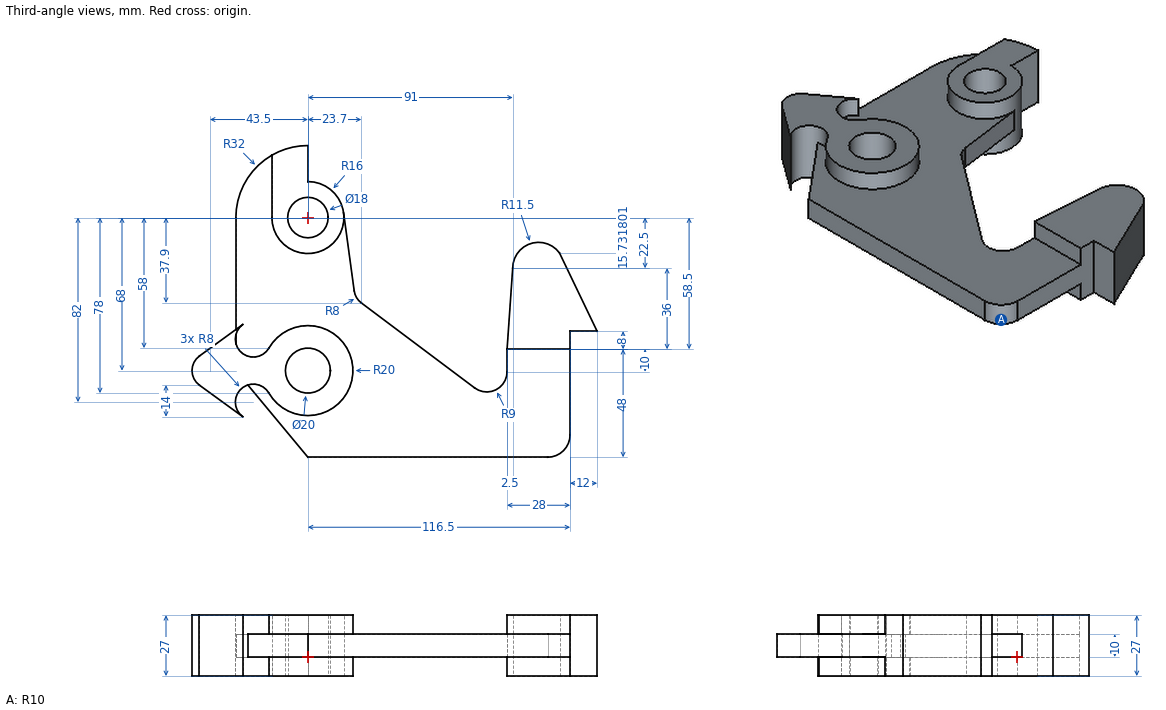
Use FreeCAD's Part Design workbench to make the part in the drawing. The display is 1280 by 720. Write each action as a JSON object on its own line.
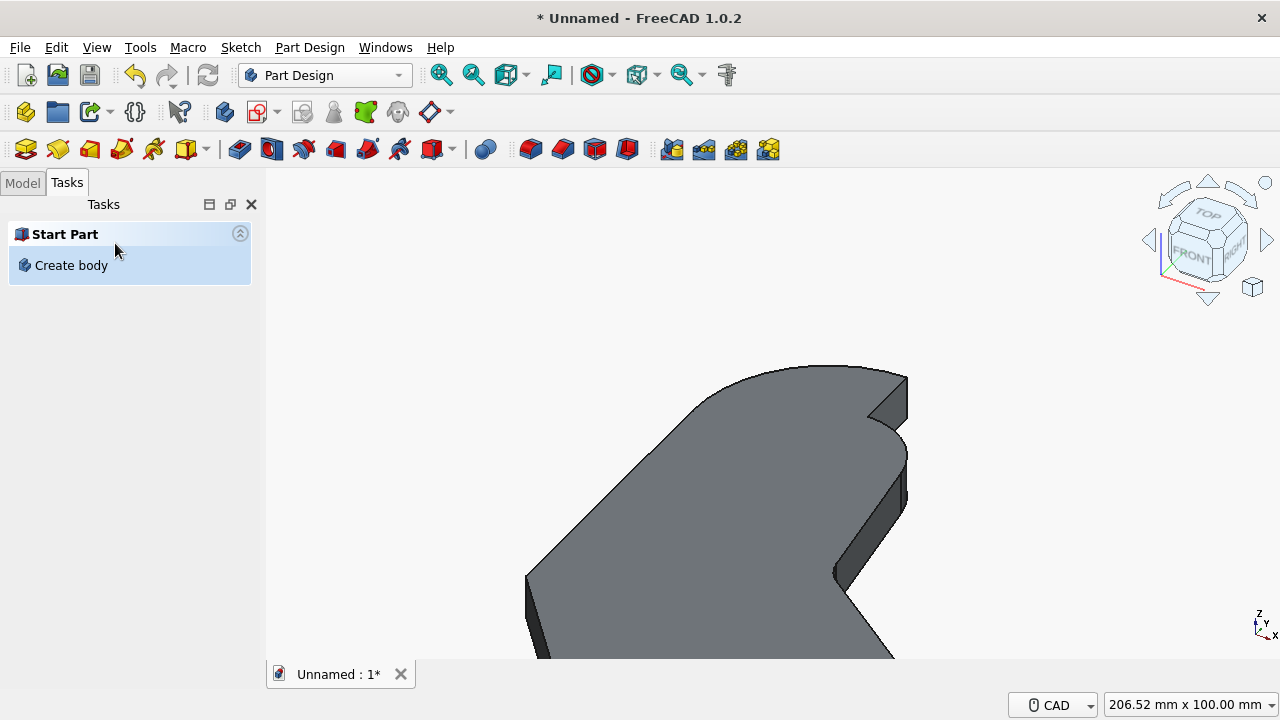
{"action": "left_click", "coordinate": [442, 76]}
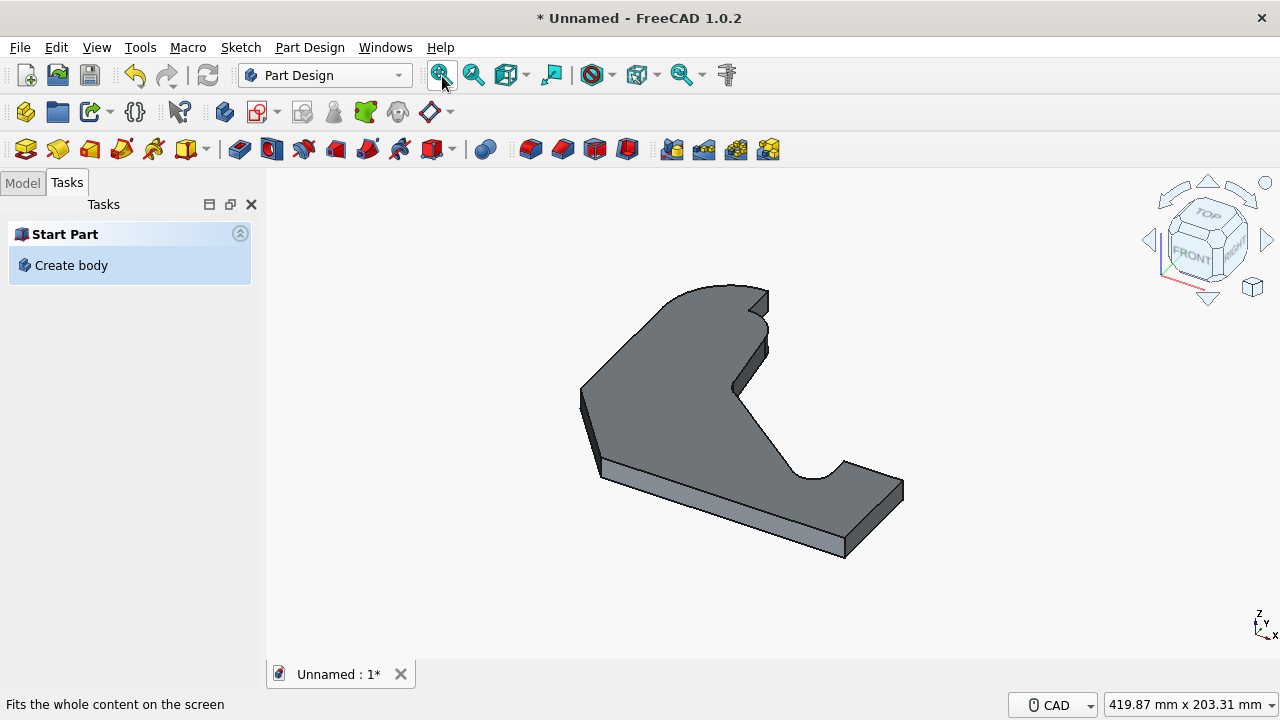
{"action": "left_click", "coordinate": [23, 182]}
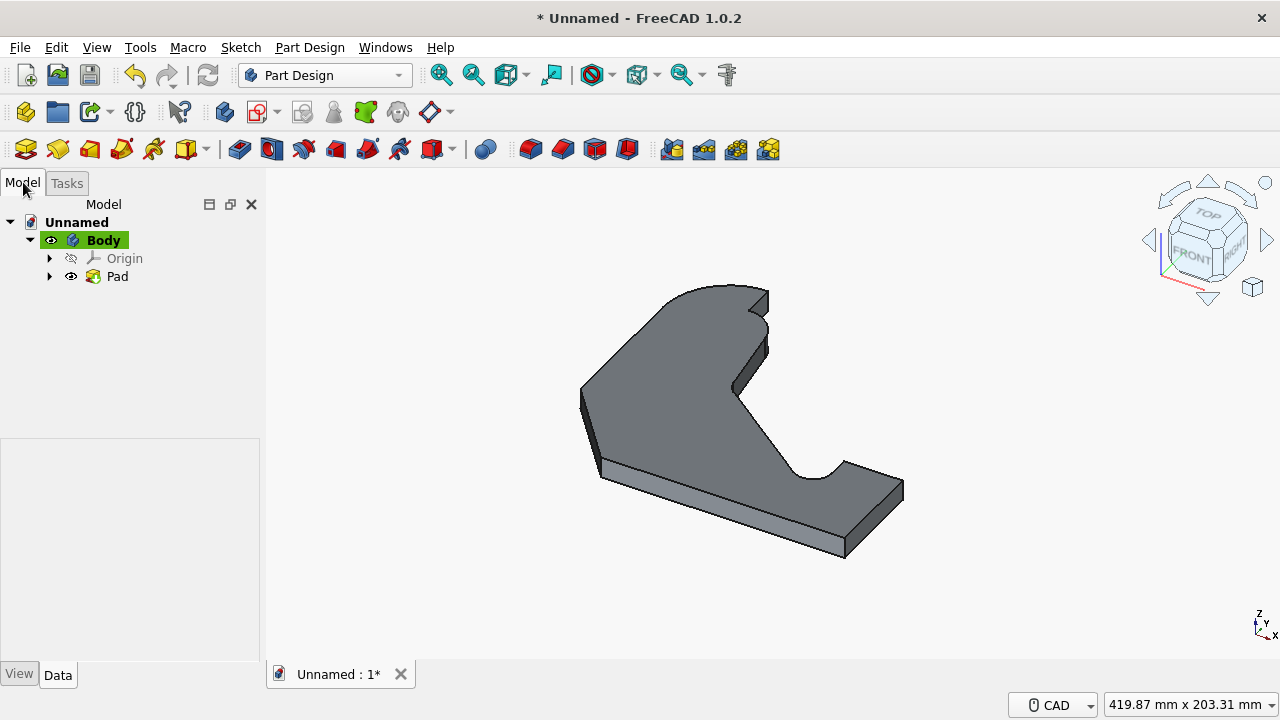
{"action": "left_click", "coordinate": [50, 258]}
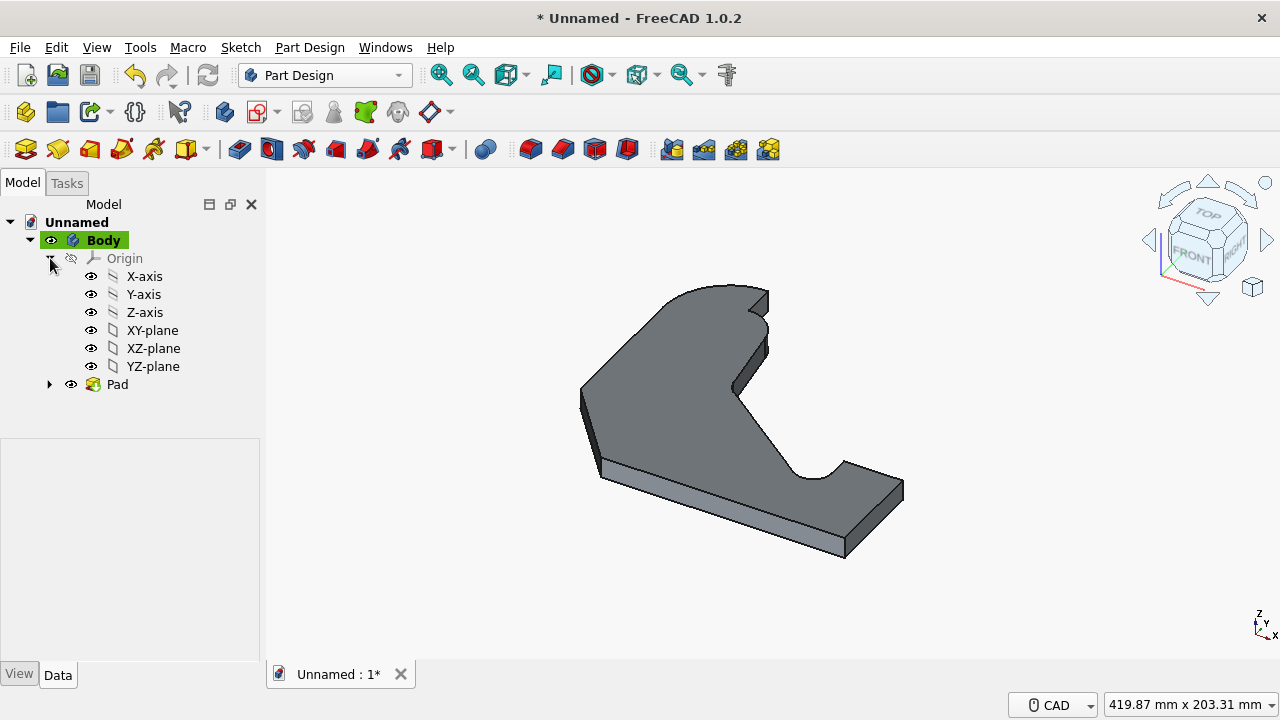
{"action": "left_click", "coordinate": [136, 330]}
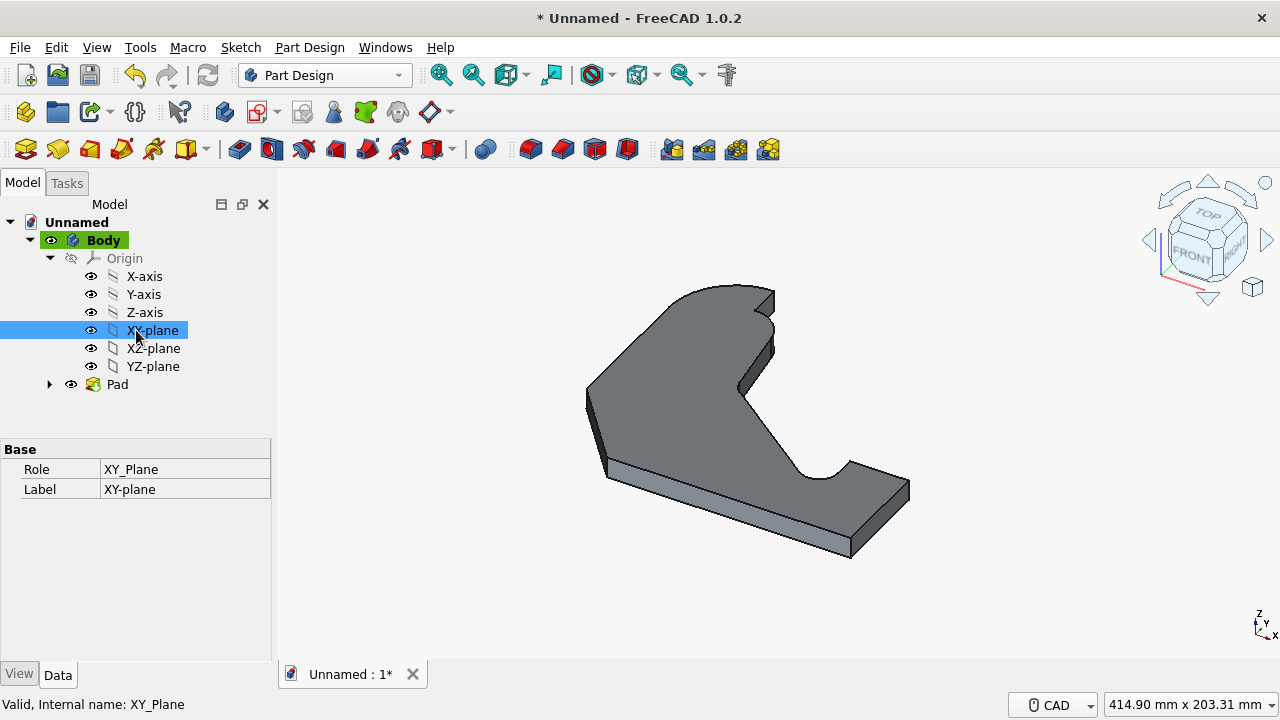
{"action": "left_click", "coordinate": [430, 112]}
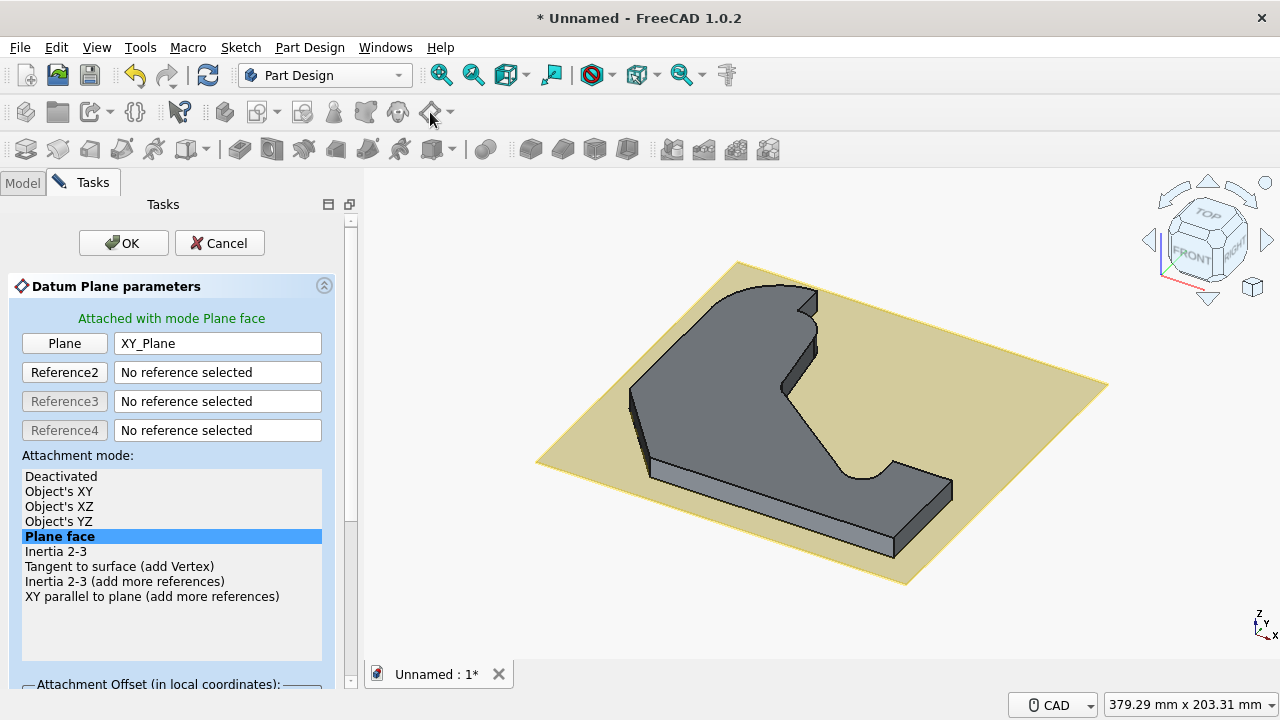
{"action": "scroll", "coordinate": [351, 451], "scroll_direction": "down", "scroll_amount": 3}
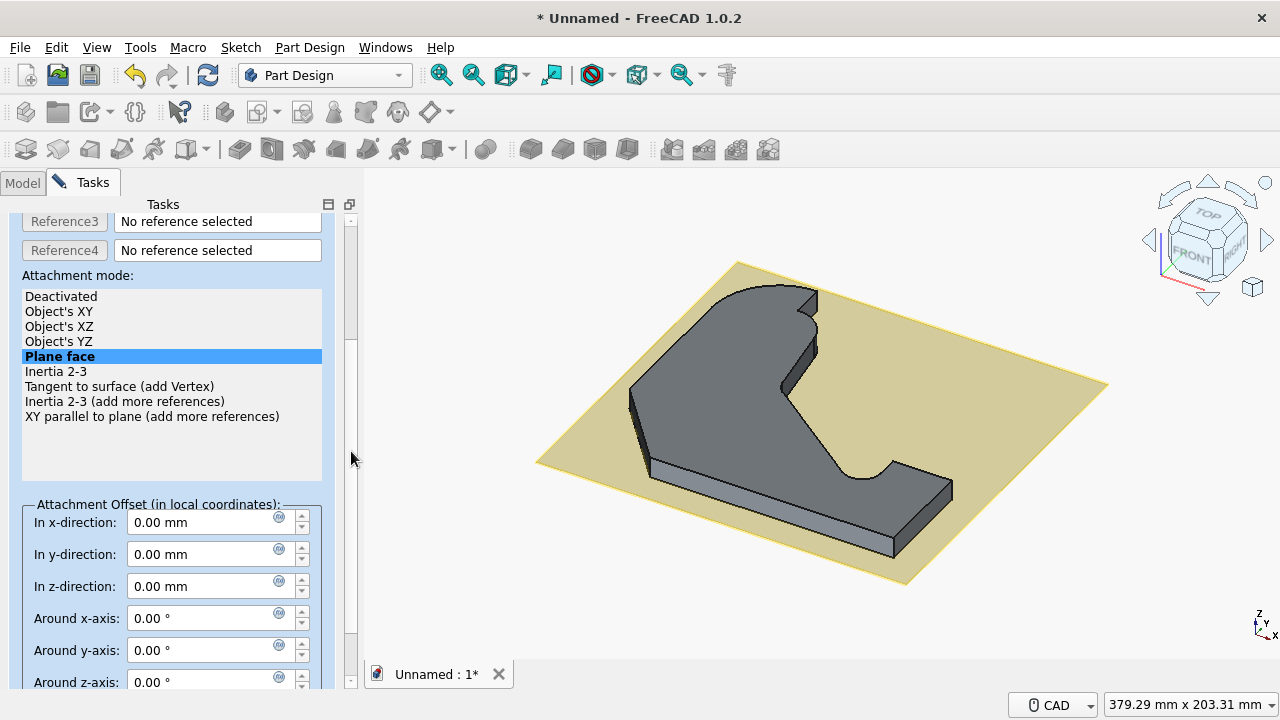
{"action": "triple_click", "coordinate": [210, 586]}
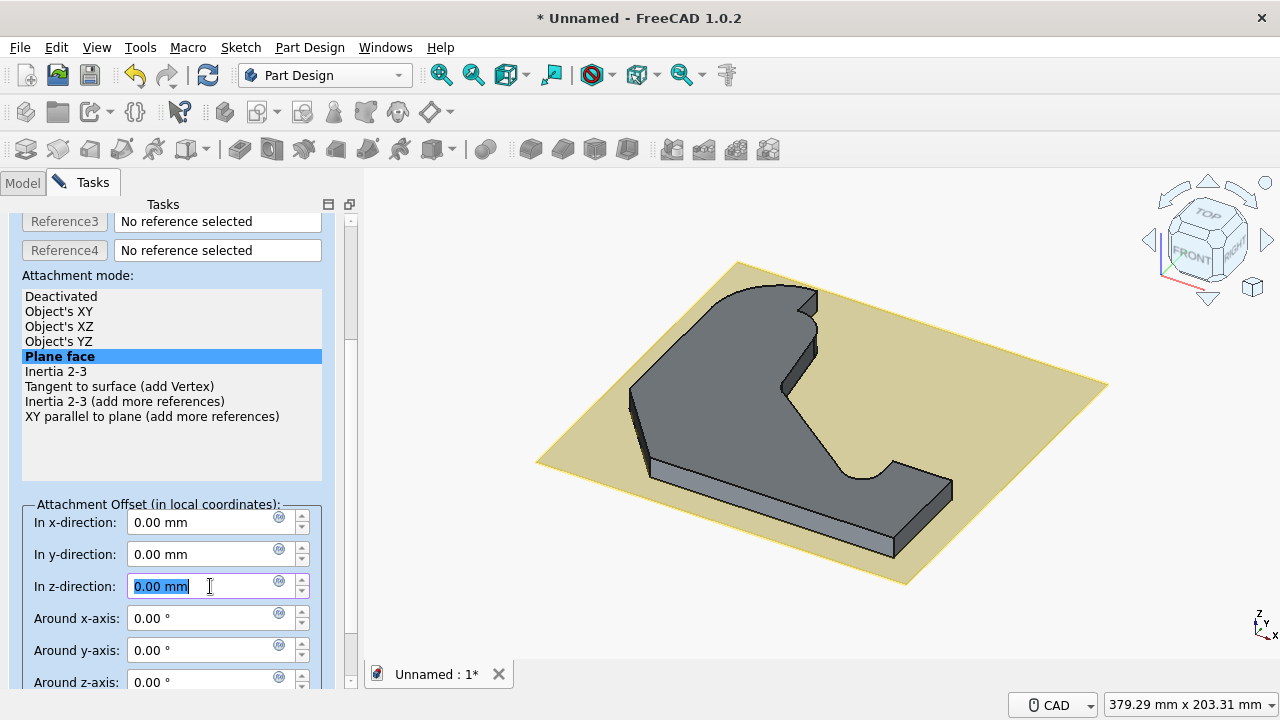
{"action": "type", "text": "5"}
{"action": "key", "text": "Tab"}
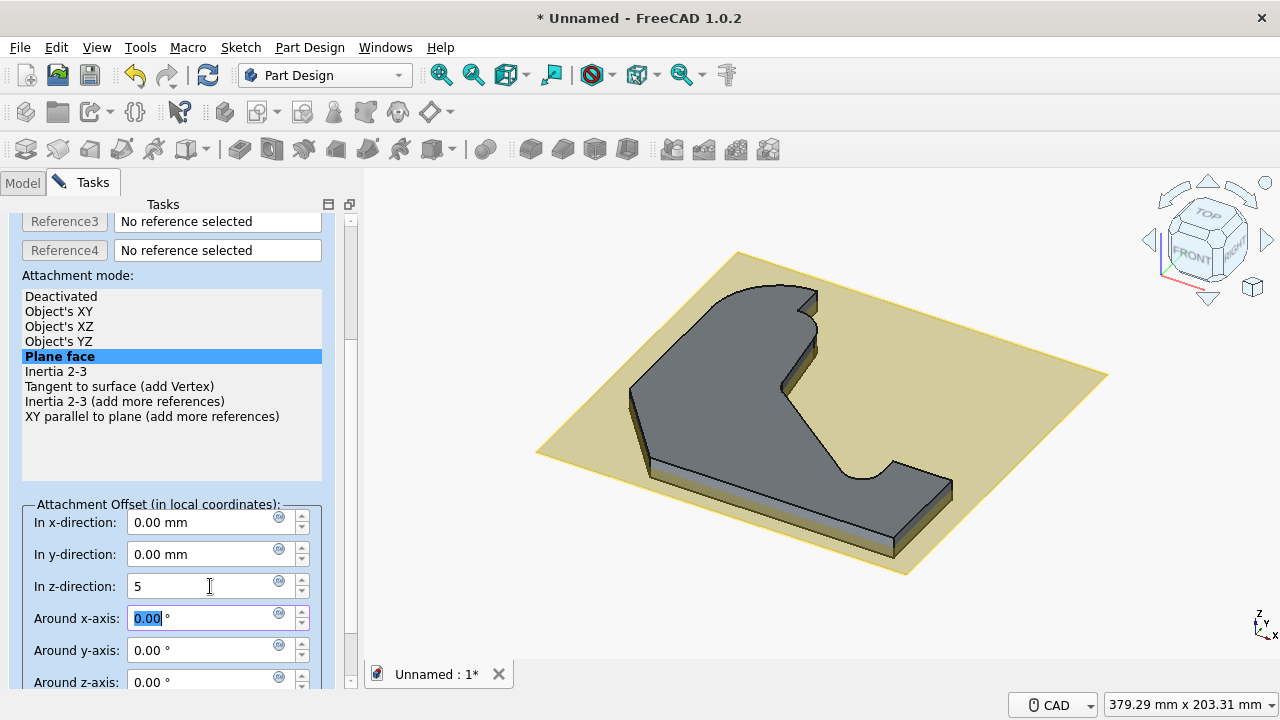
{"action": "scroll", "coordinate": [351, 451], "scroll_direction": "up", "scroll_amount": 4}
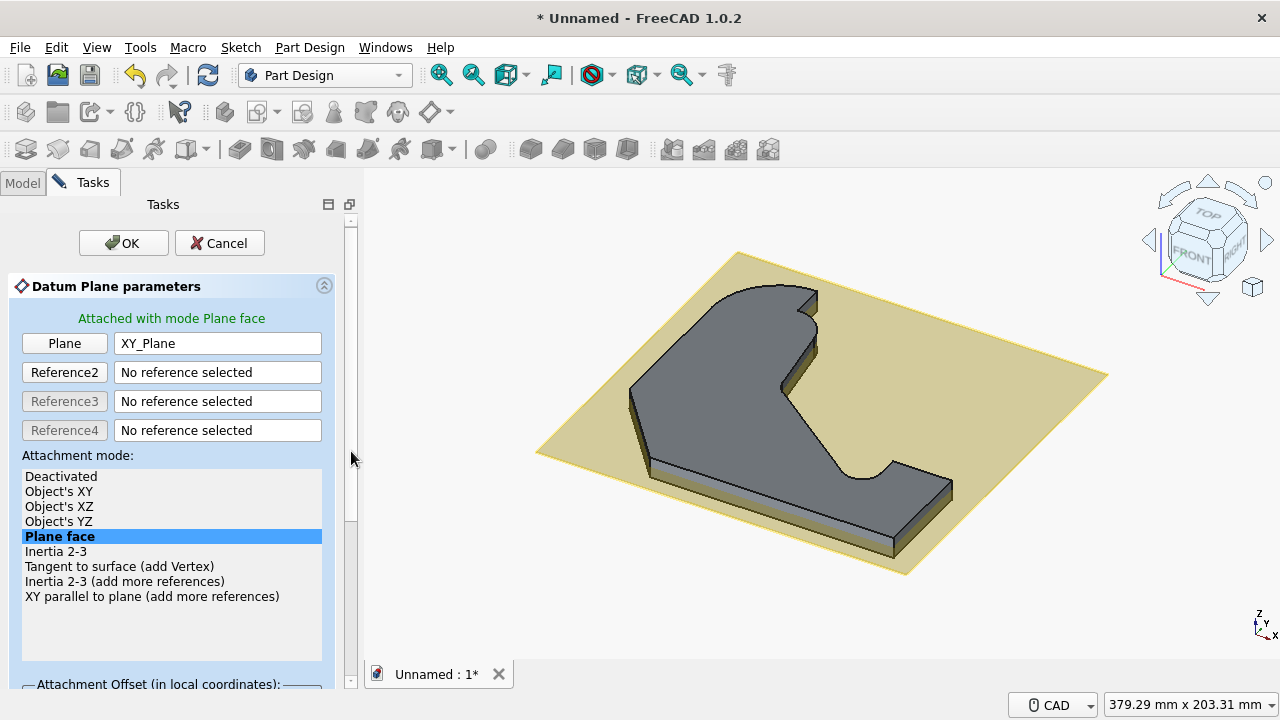
{"action": "left_click", "coordinate": [124, 243]}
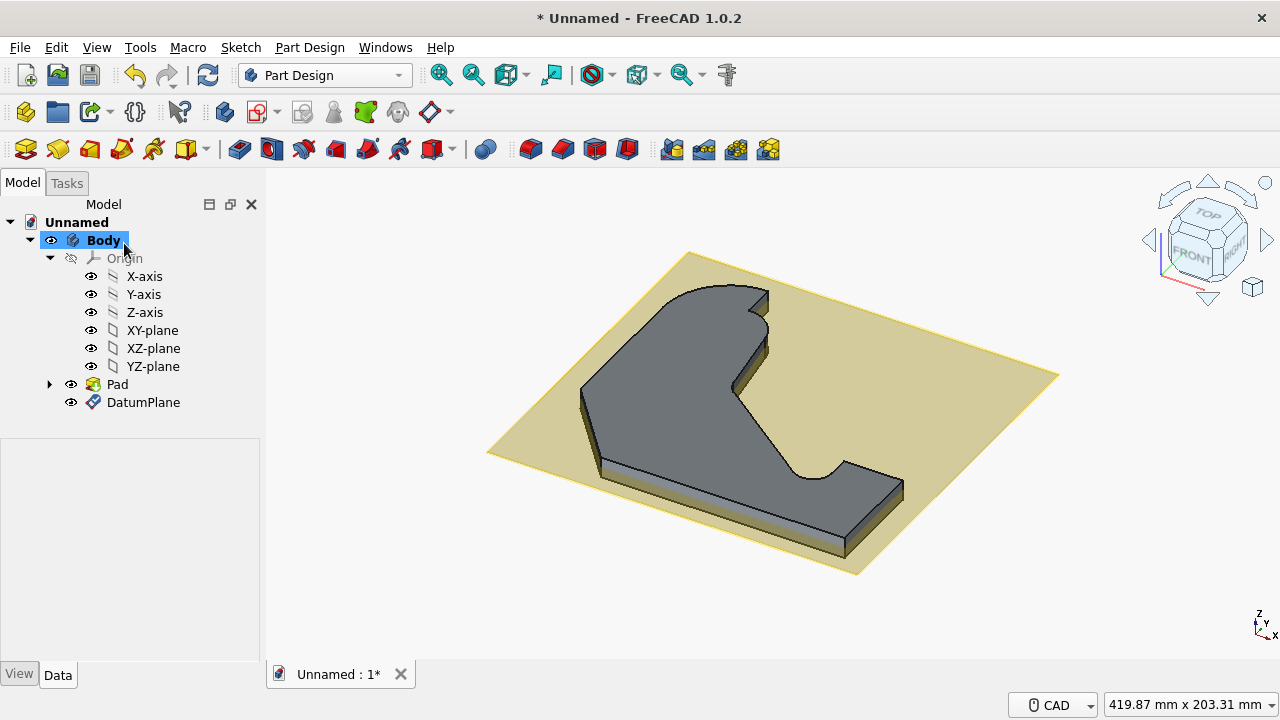
{"action": "left_click", "coordinate": [116, 402]}